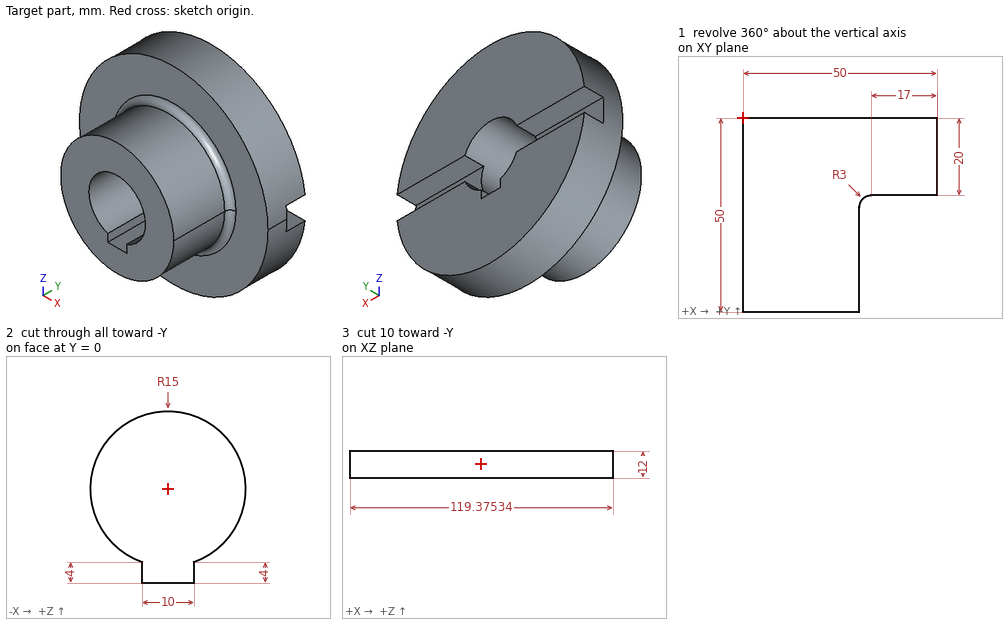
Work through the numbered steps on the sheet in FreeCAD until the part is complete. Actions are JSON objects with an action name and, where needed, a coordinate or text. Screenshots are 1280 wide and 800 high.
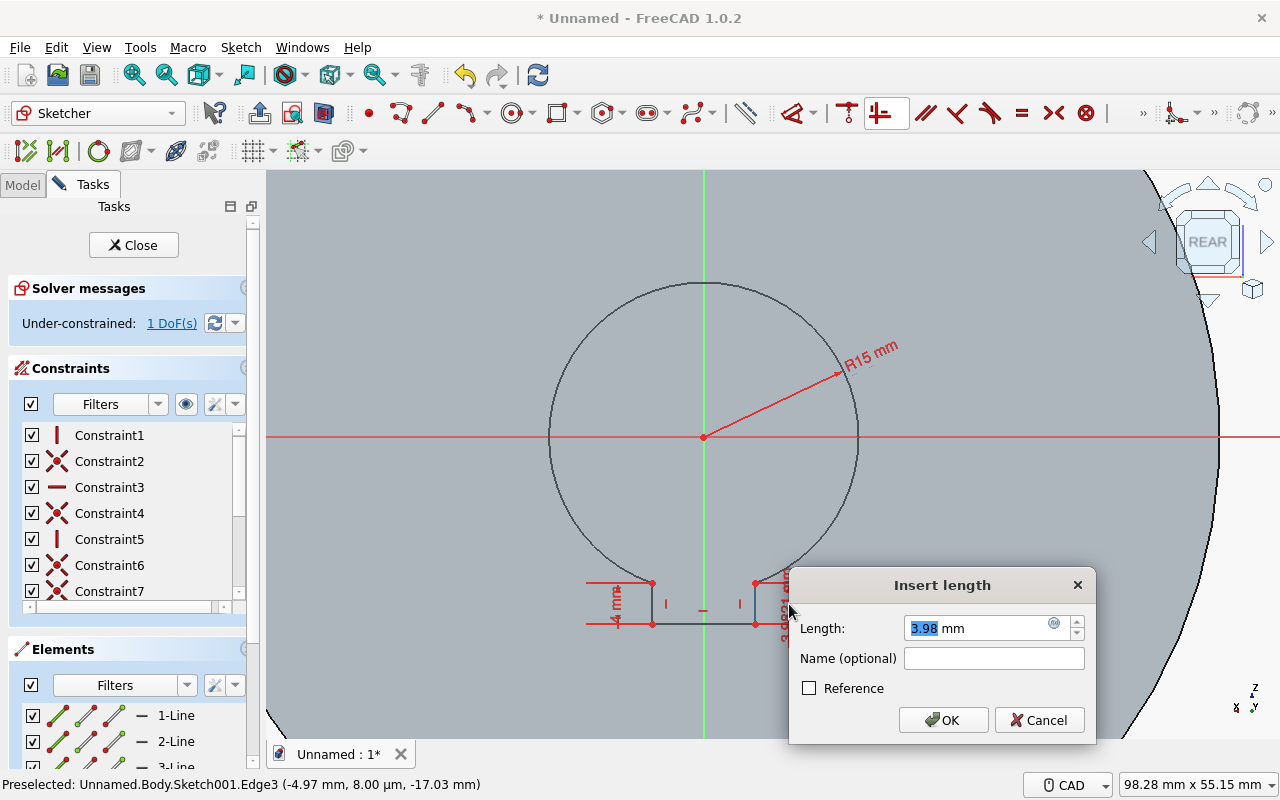
{"action": "type", "text": "4"}
{"action": "key", "text": "Return"}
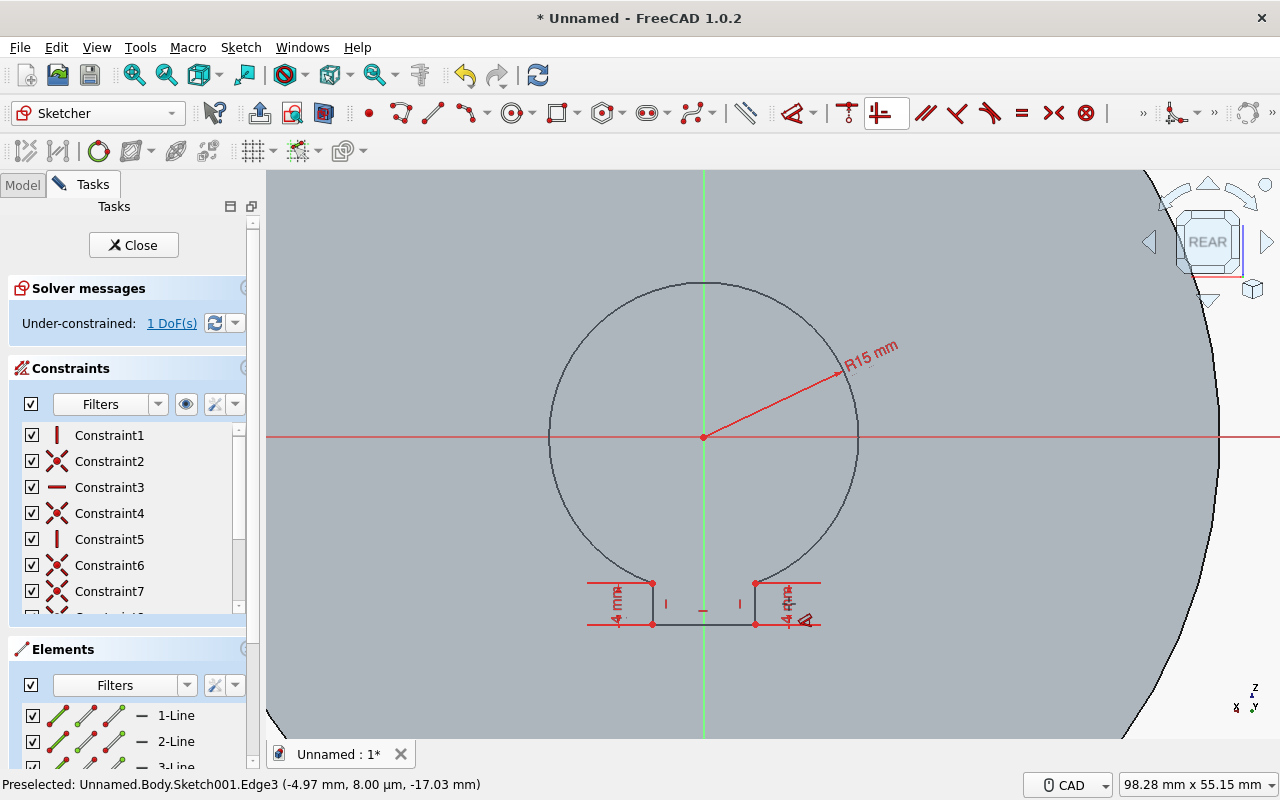
{"action": "left_click", "coordinate": [683, 625]}
{"action": "left_click", "coordinate": [680, 659]}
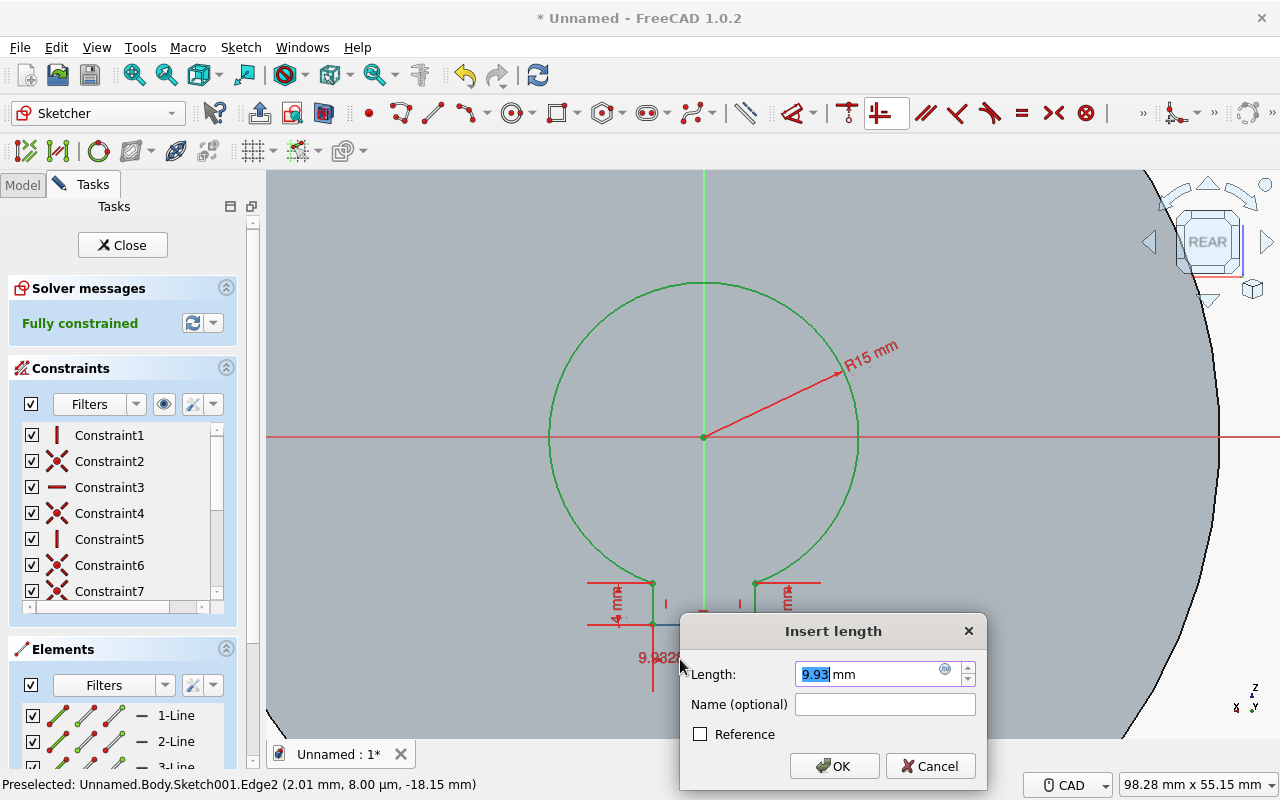
{"action": "type", "text": "10"}
{"action": "key", "text": "Return"}
{"action": "key", "text": "Escape"}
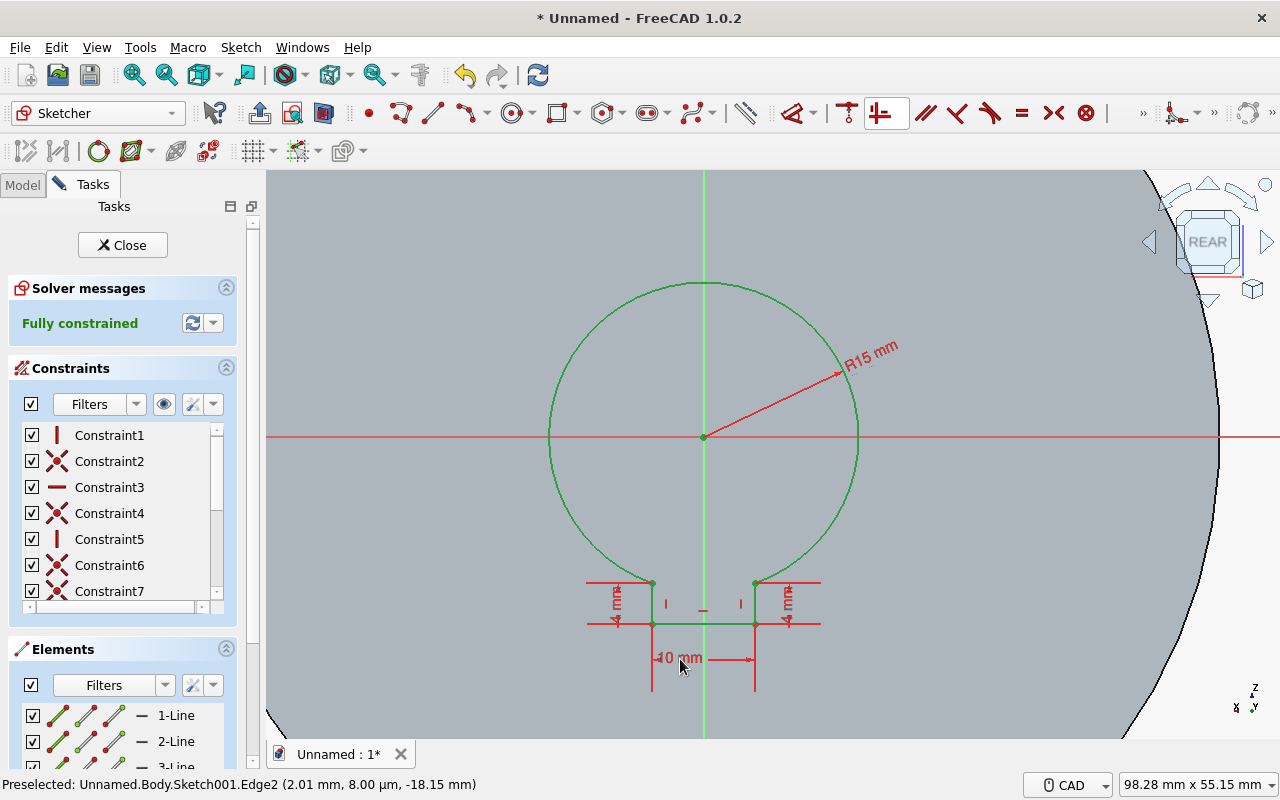
{"action": "left_click", "coordinate": [123, 245]}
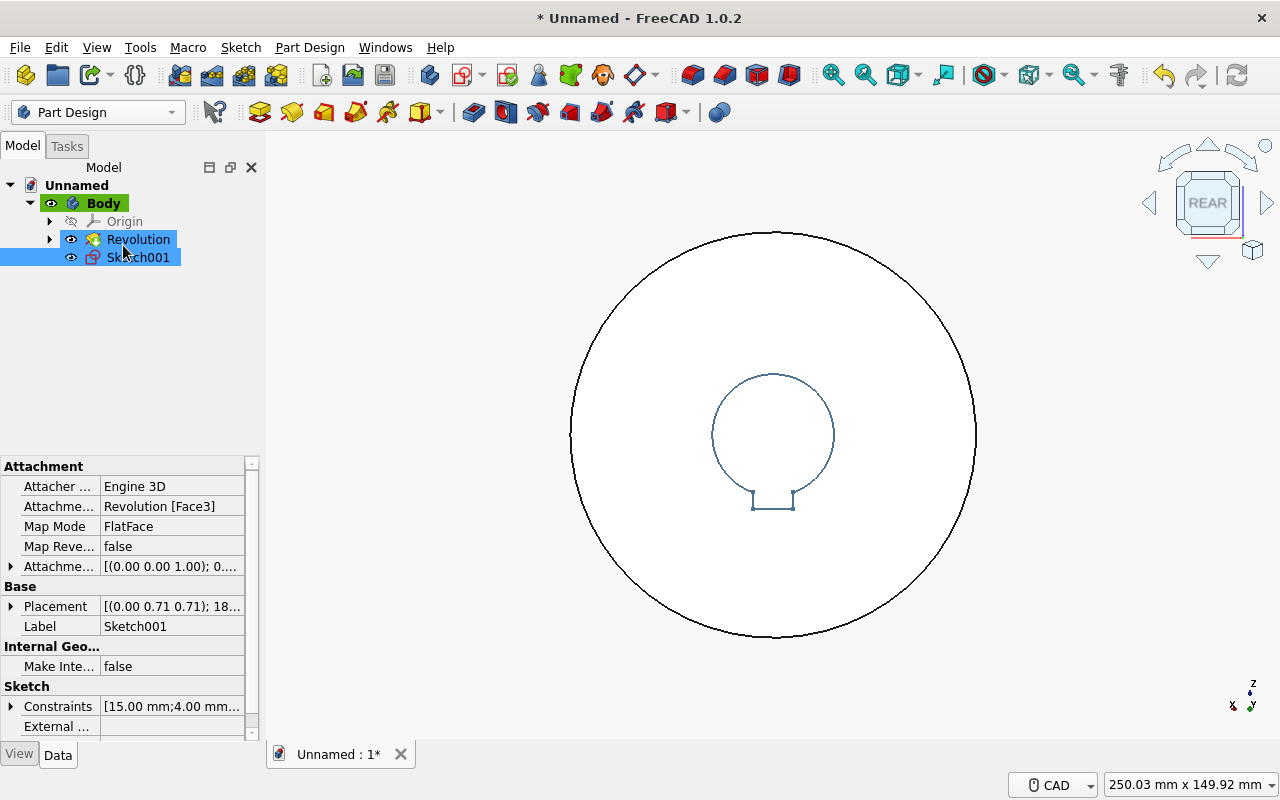
{"action": "left_click", "coordinate": [474, 112]}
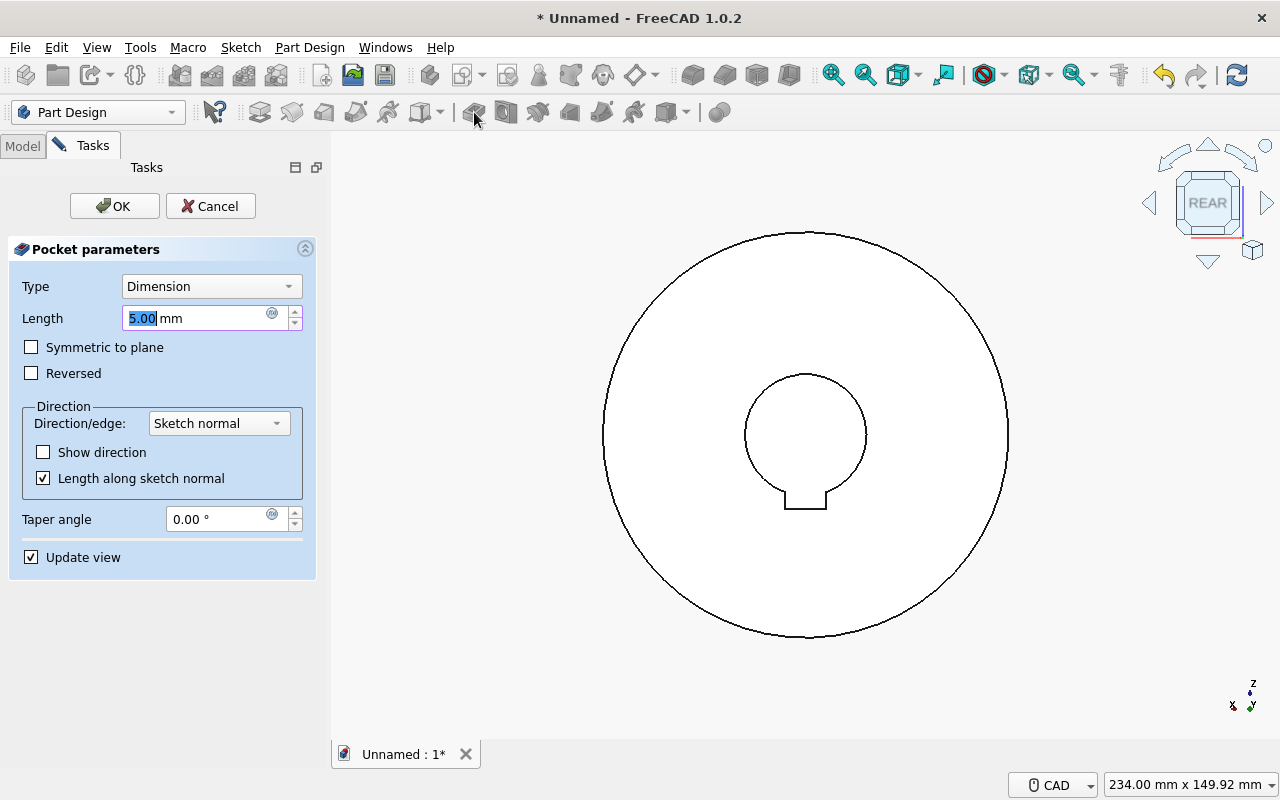
{"action": "left_click", "coordinate": [212, 286]}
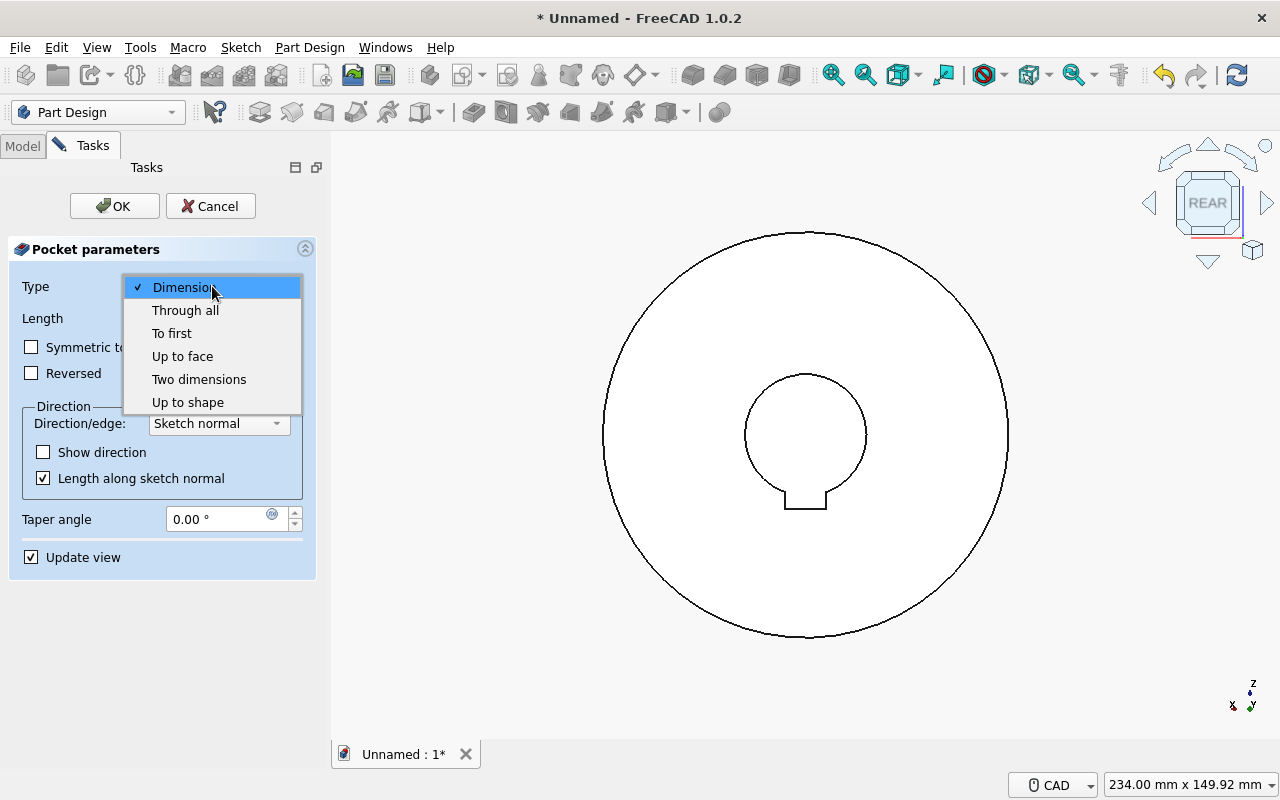
{"action": "left_click", "coordinate": [212, 310]}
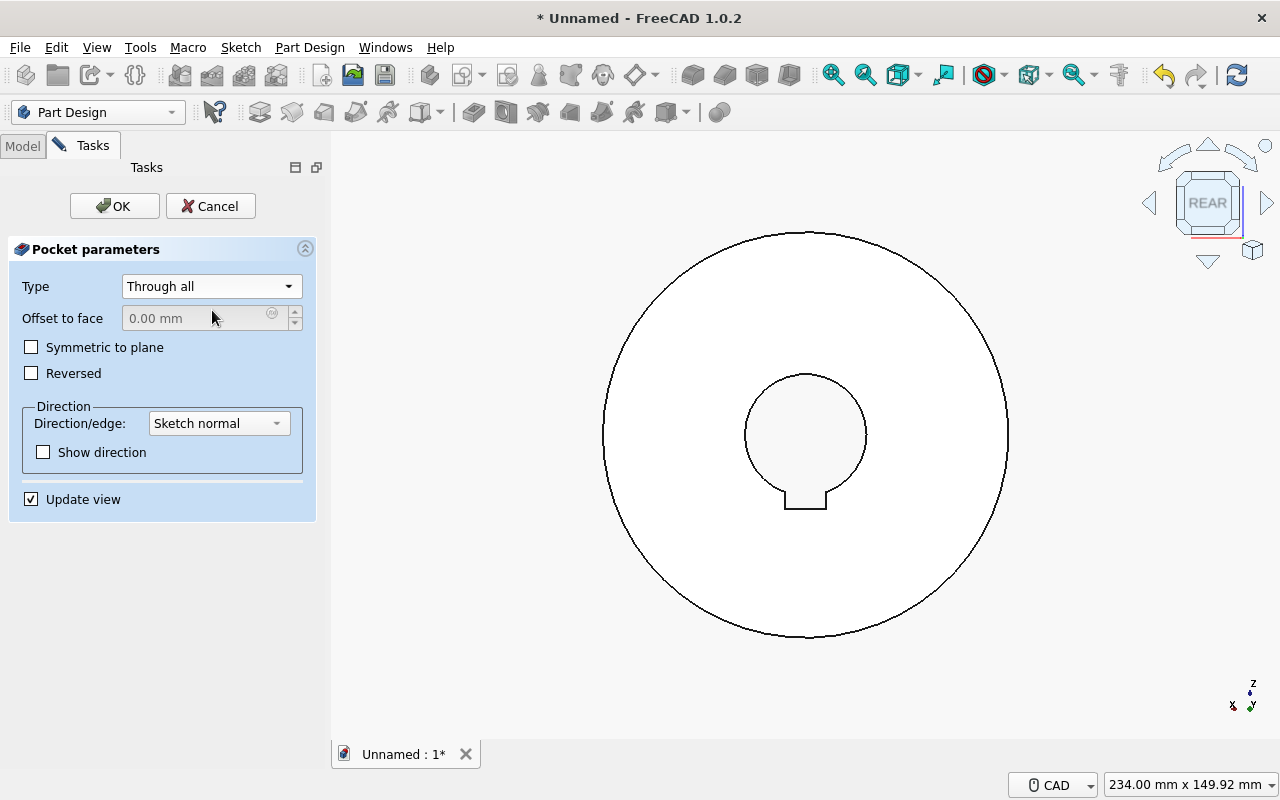
{"action": "left_click", "coordinate": [115, 206]}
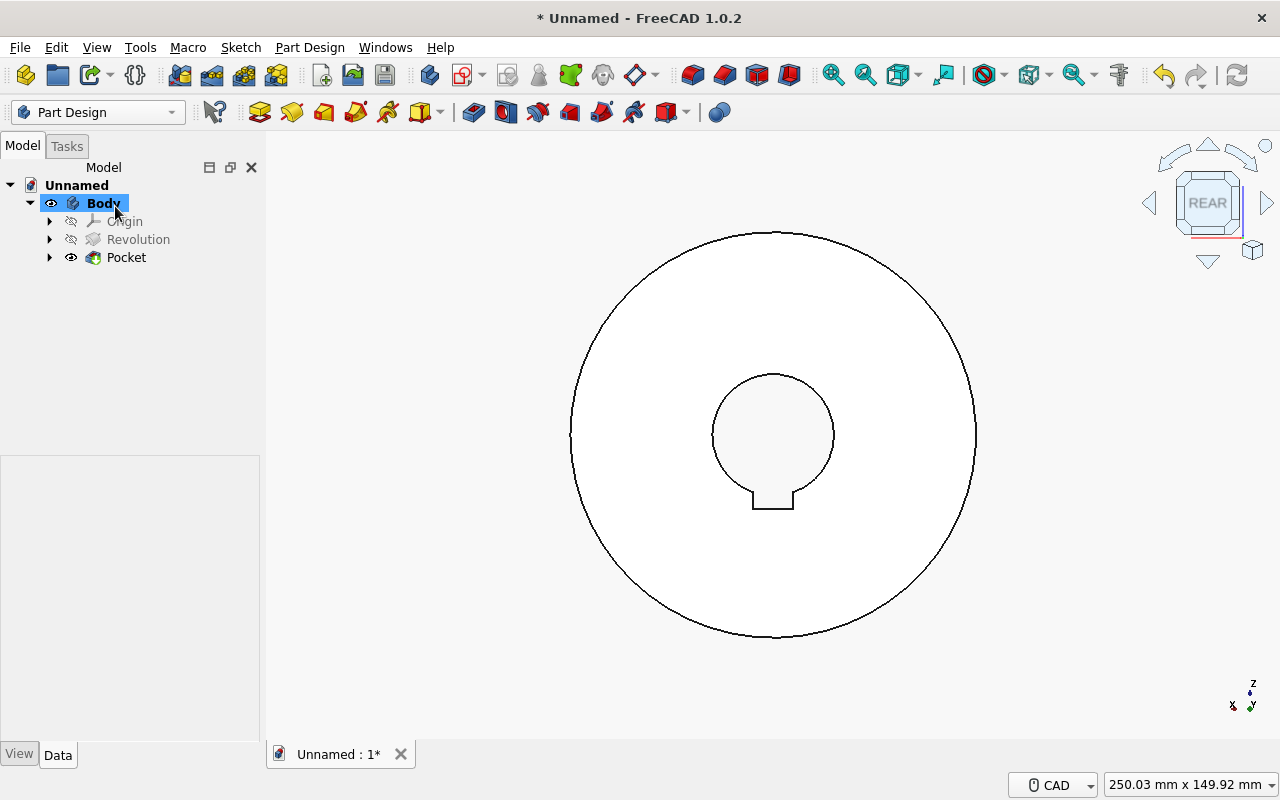
{"action": "left_click", "coordinate": [462, 76]}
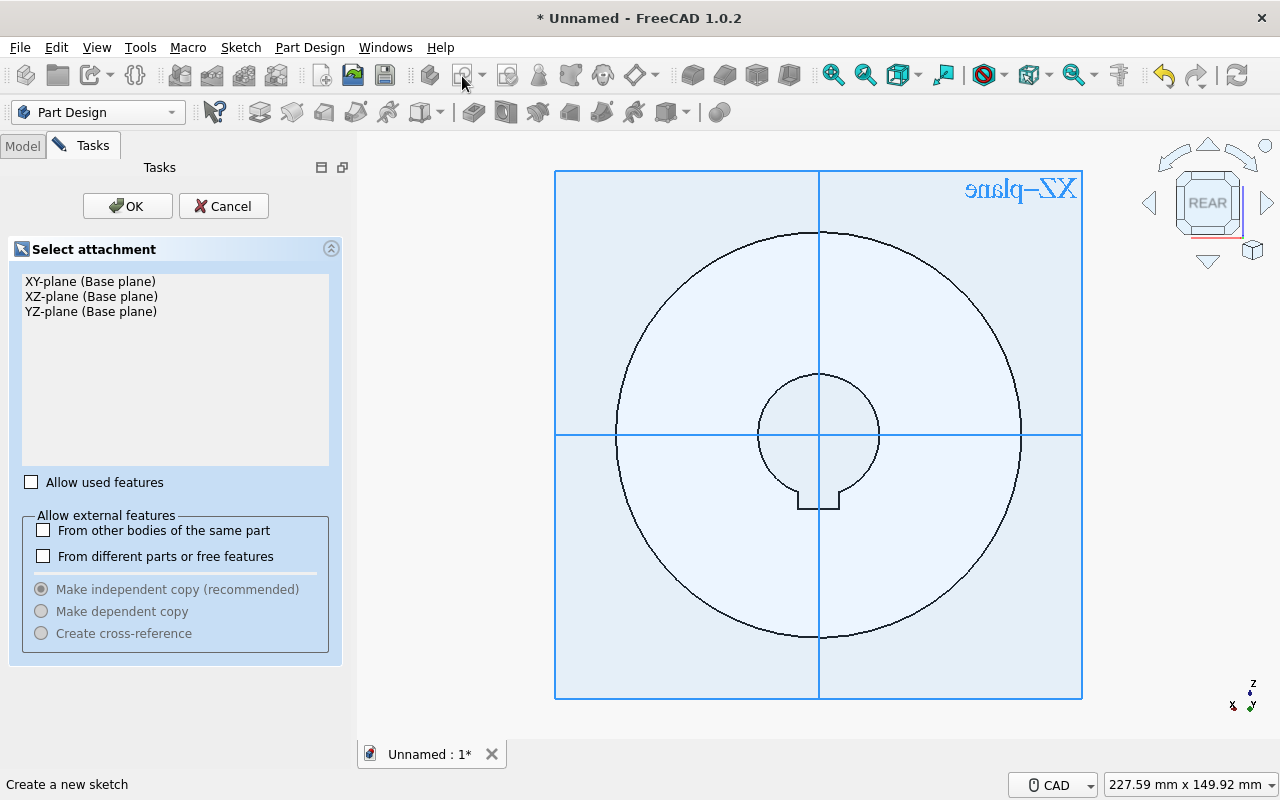
{"action": "left_click", "coordinate": [82, 296]}